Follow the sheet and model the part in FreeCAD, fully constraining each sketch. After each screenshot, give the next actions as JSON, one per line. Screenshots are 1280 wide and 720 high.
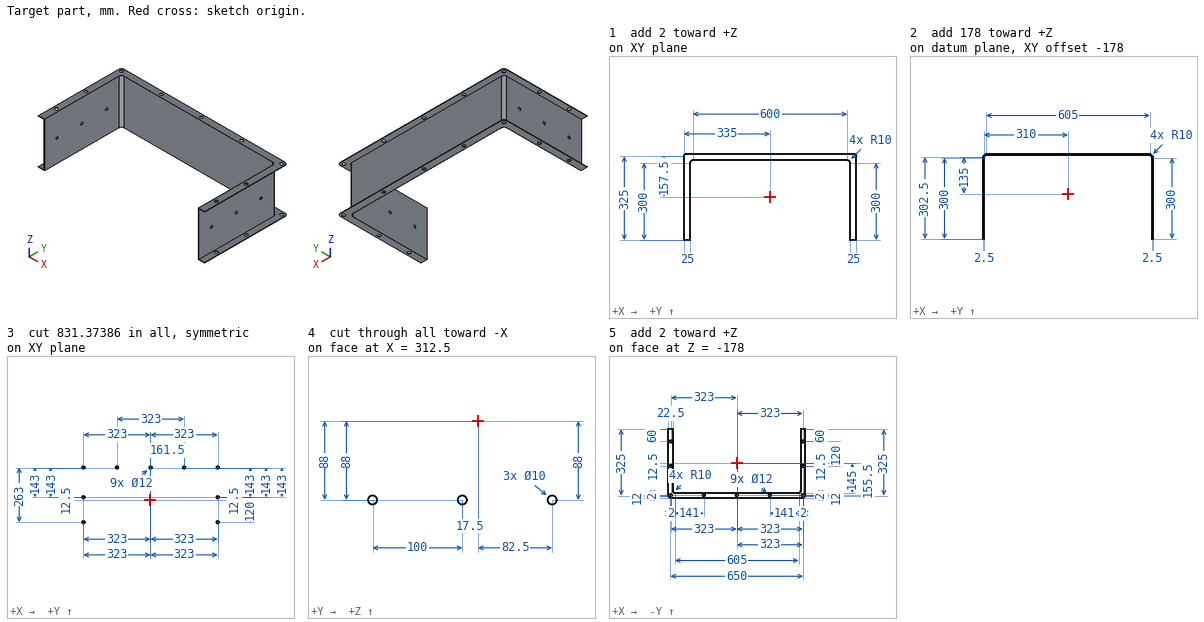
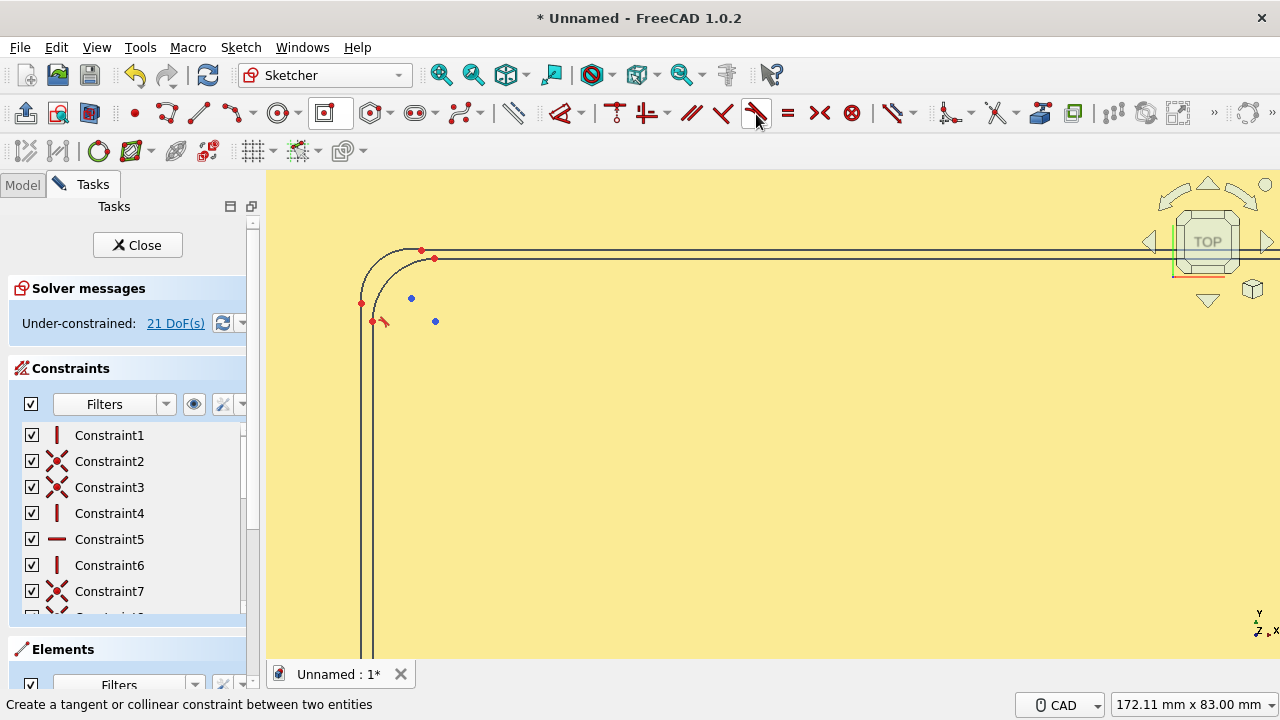
{"action": "scroll", "coordinate": [408, 266], "scroll_direction": "down", "scroll_amount": 9}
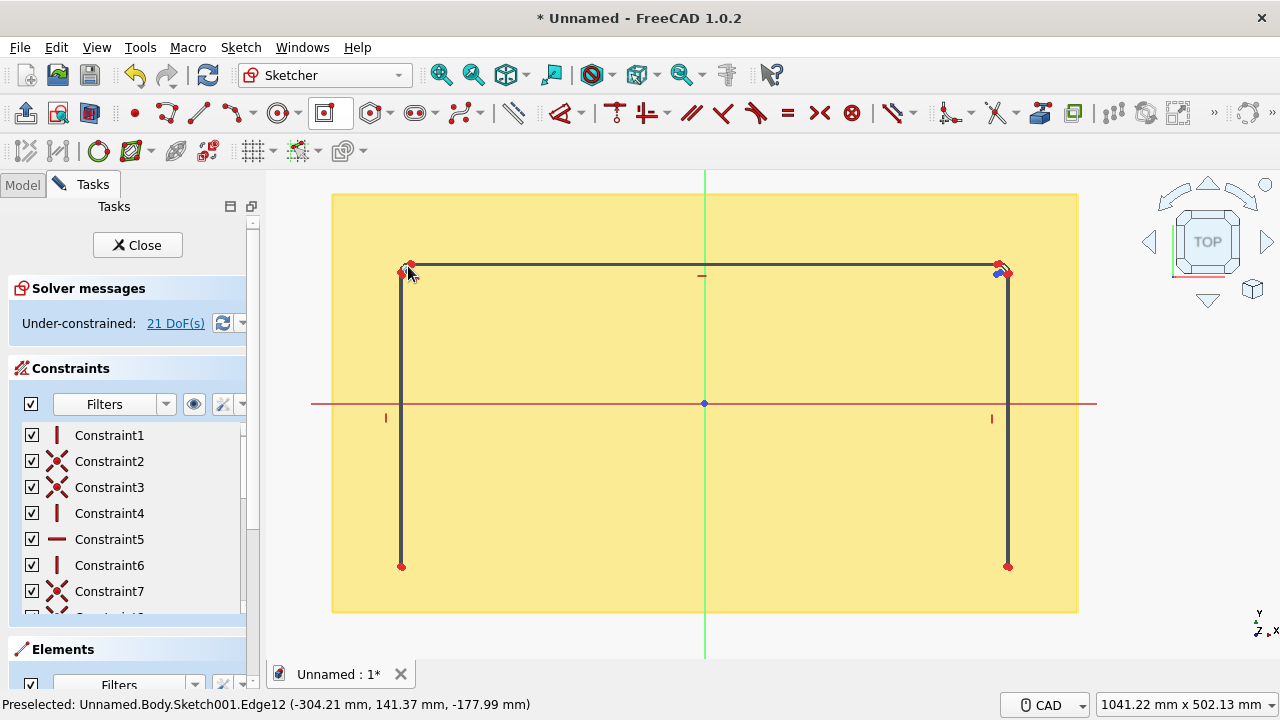
{"action": "scroll", "coordinate": [400, 478], "scroll_direction": "up", "scroll_amount": 10}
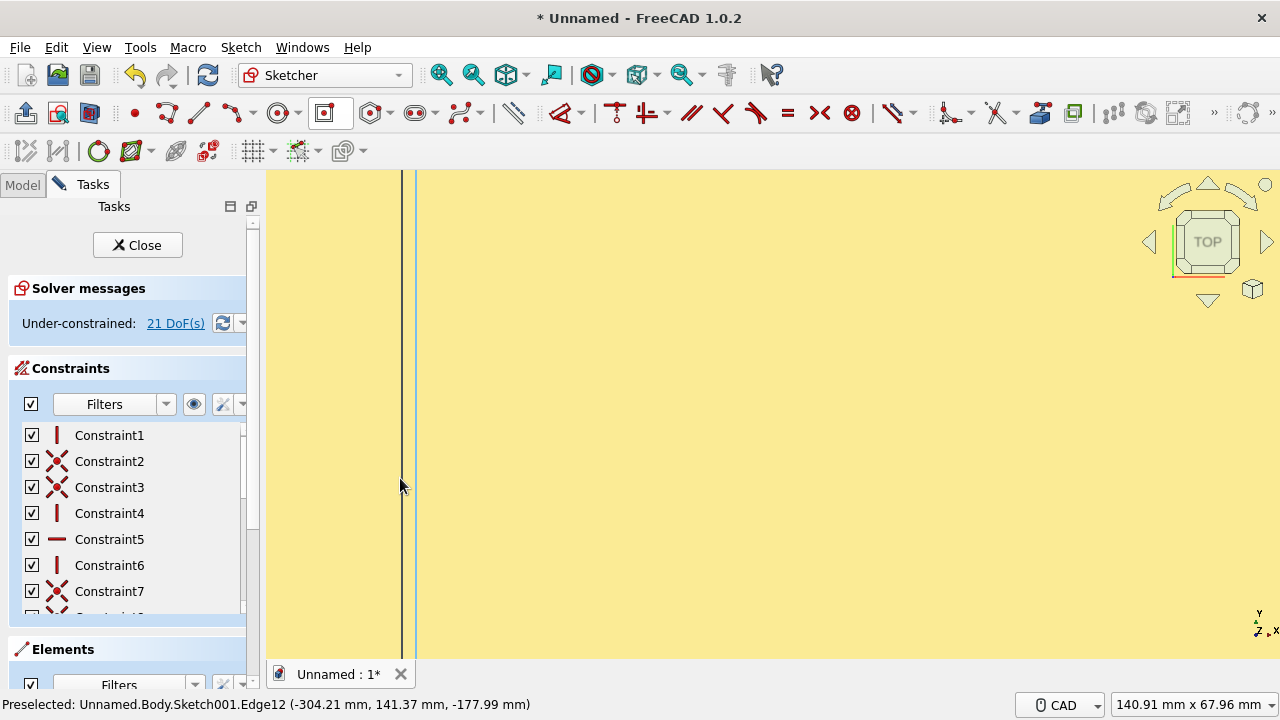
{"action": "left_click", "coordinate": [402, 476]}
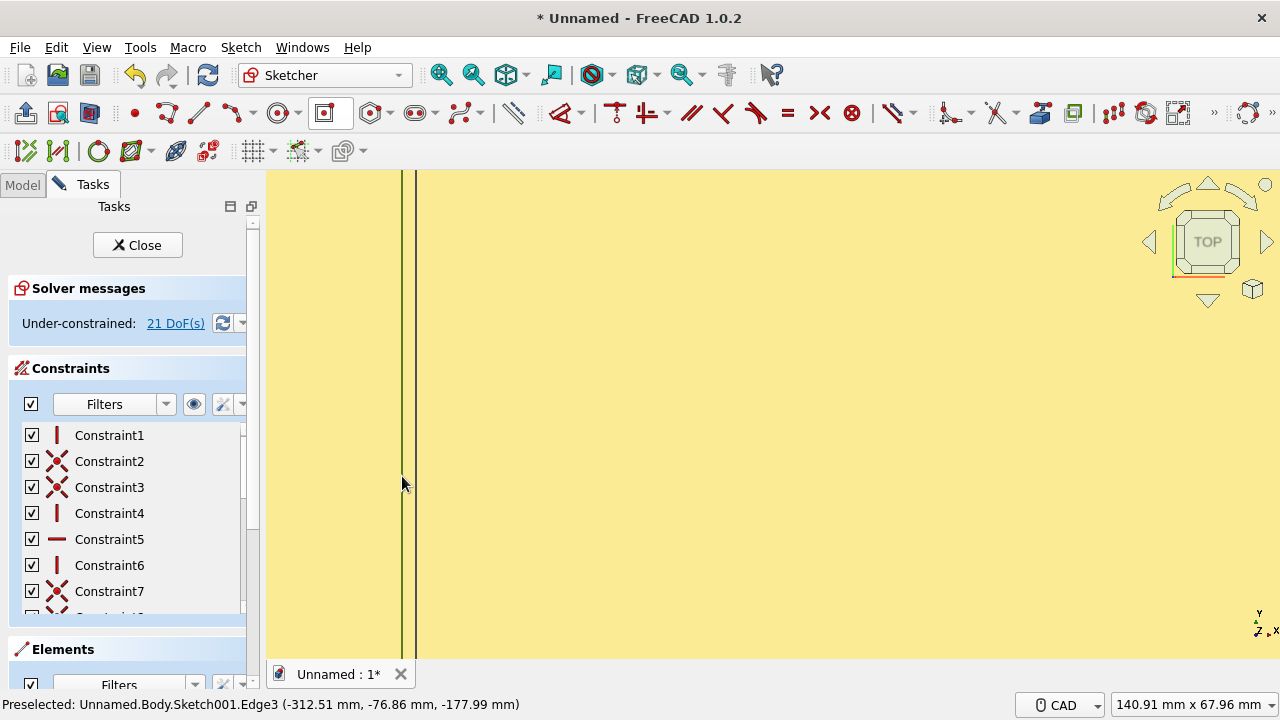
{"action": "scroll", "coordinate": [400, 479], "scroll_direction": "down", "scroll_amount": 10}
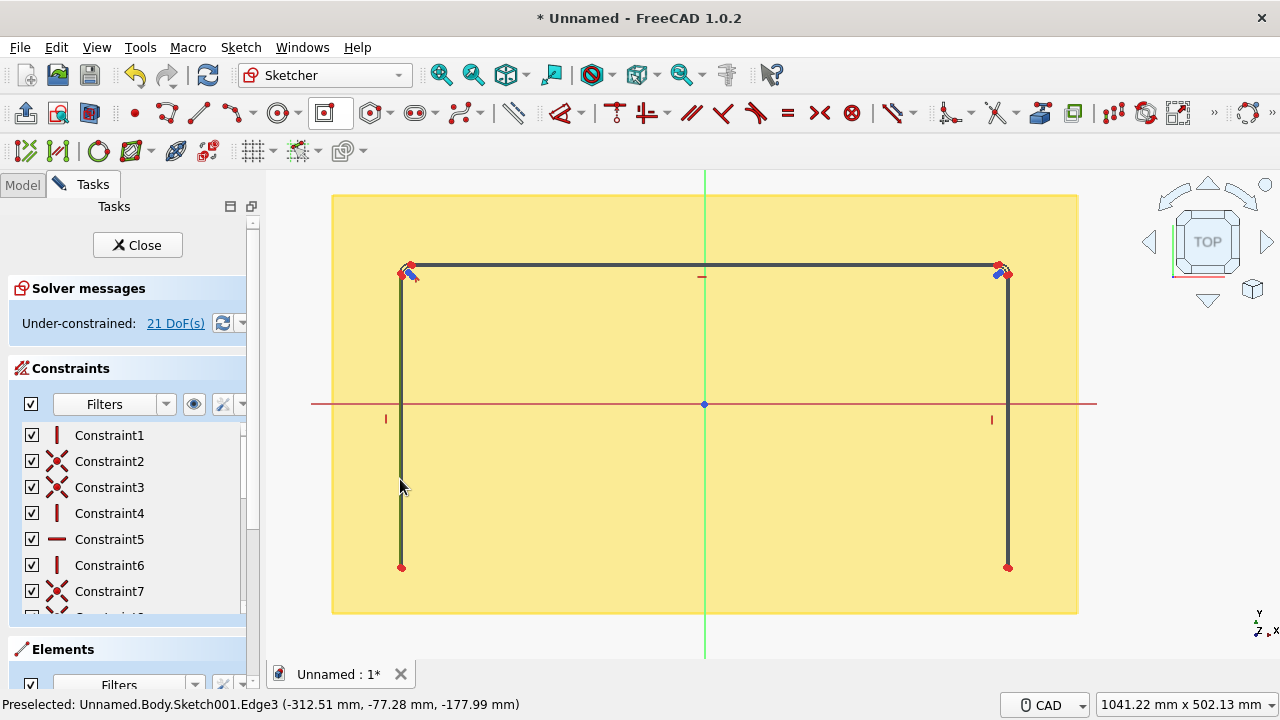
{"action": "scroll", "coordinate": [406, 265], "scroll_direction": "up", "scroll_amount": 8}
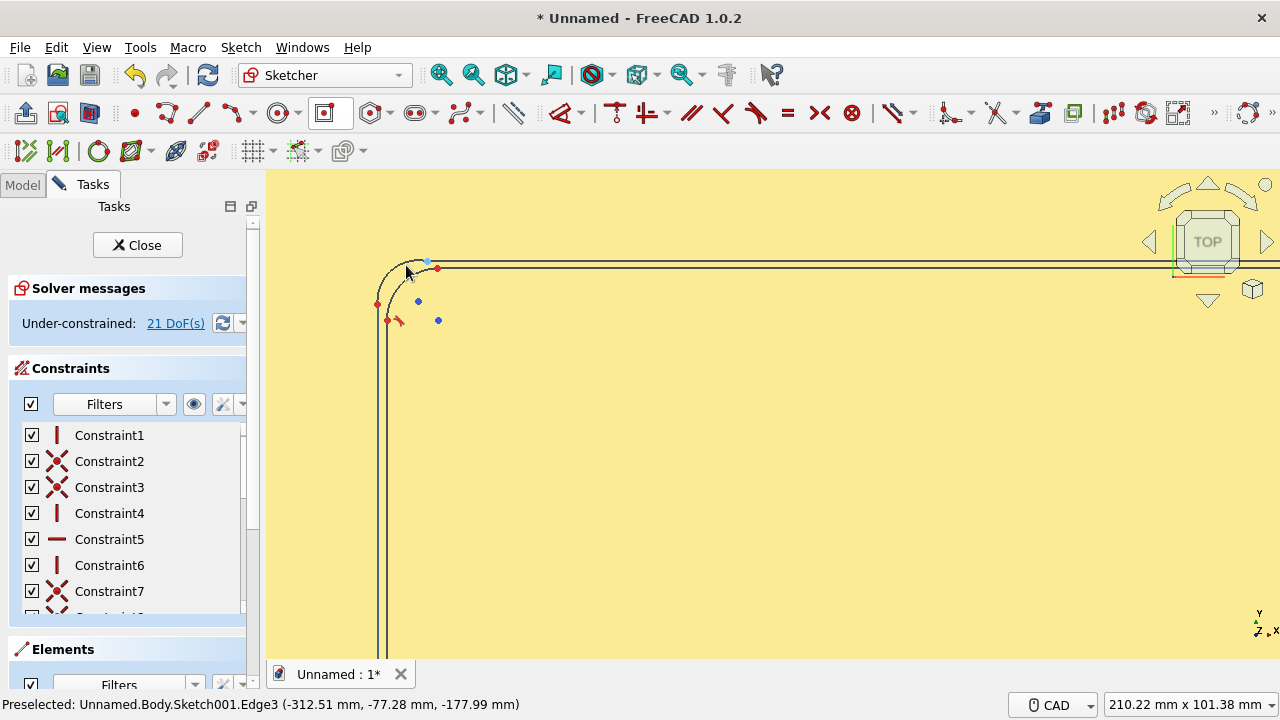
{"action": "left_click", "coordinate": [405, 263]}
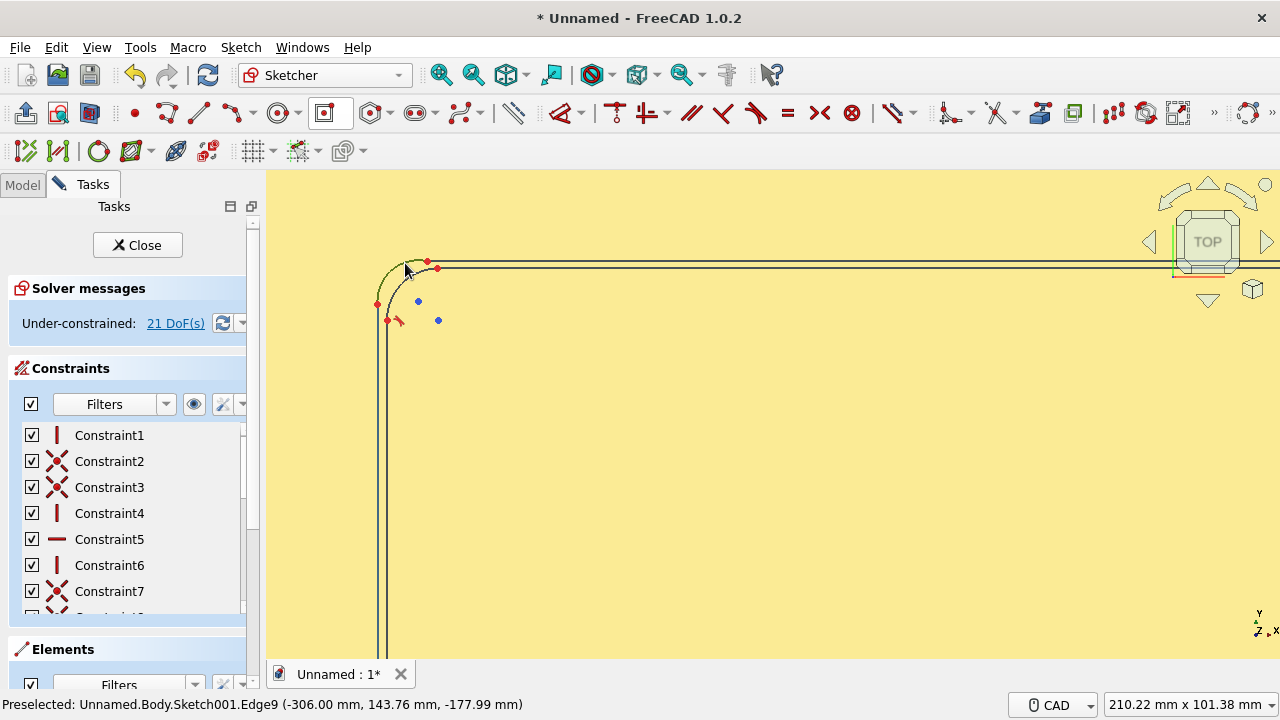
{"action": "left_click", "coordinate": [756, 114]}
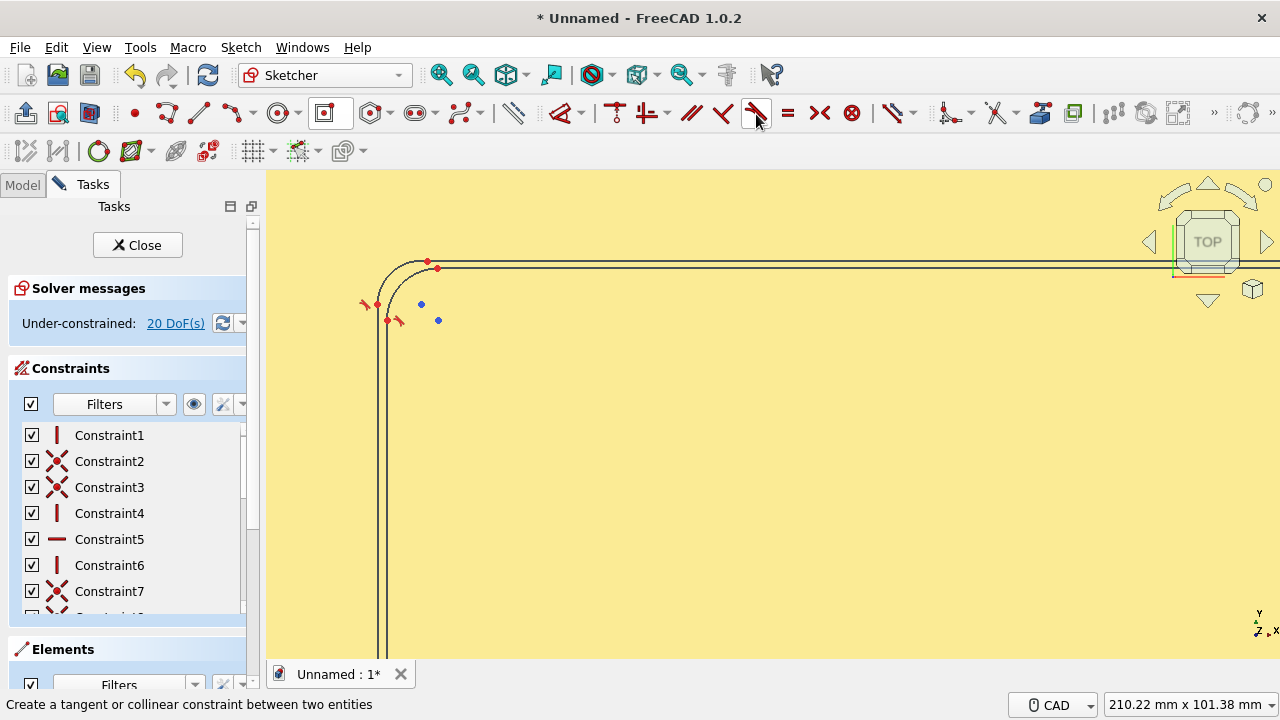
{"action": "scroll", "coordinate": [1011, 261], "scroll_direction": "up", "scroll_amount": 4}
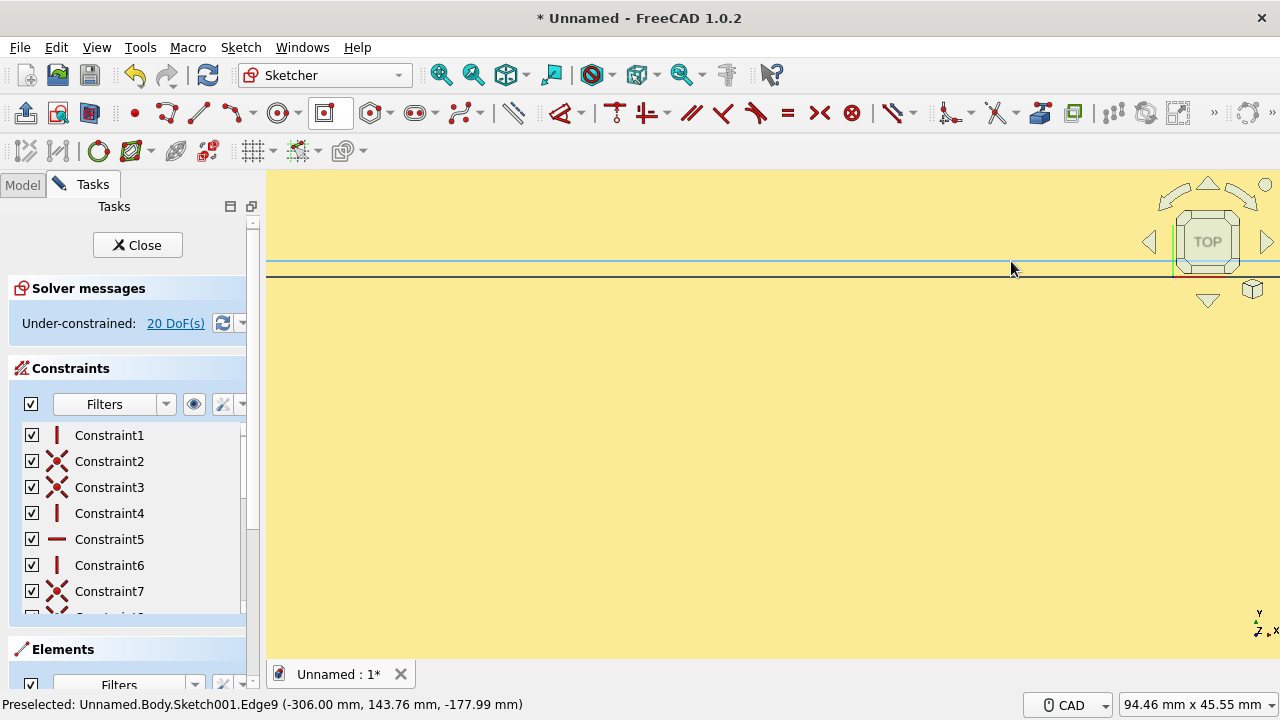
{"action": "left_click", "coordinate": [1009, 261]}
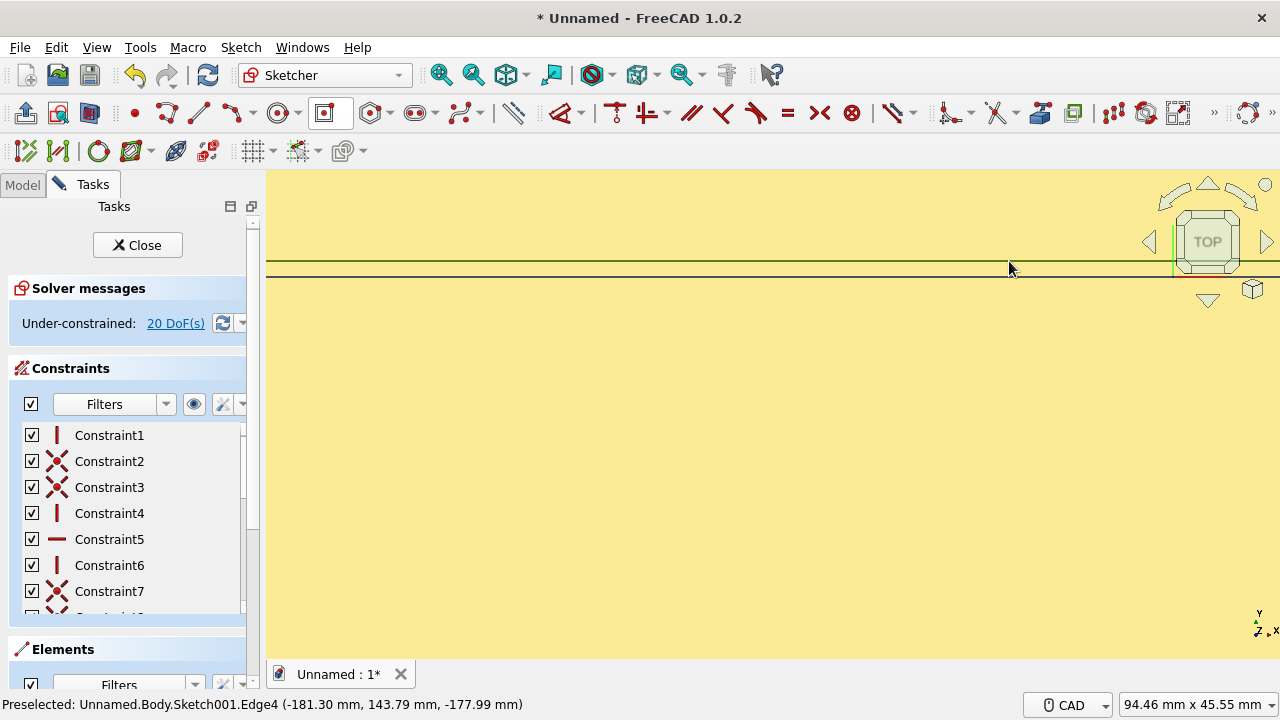
{"action": "scroll", "coordinate": [480, 264], "scroll_direction": "down", "scroll_amount": 12}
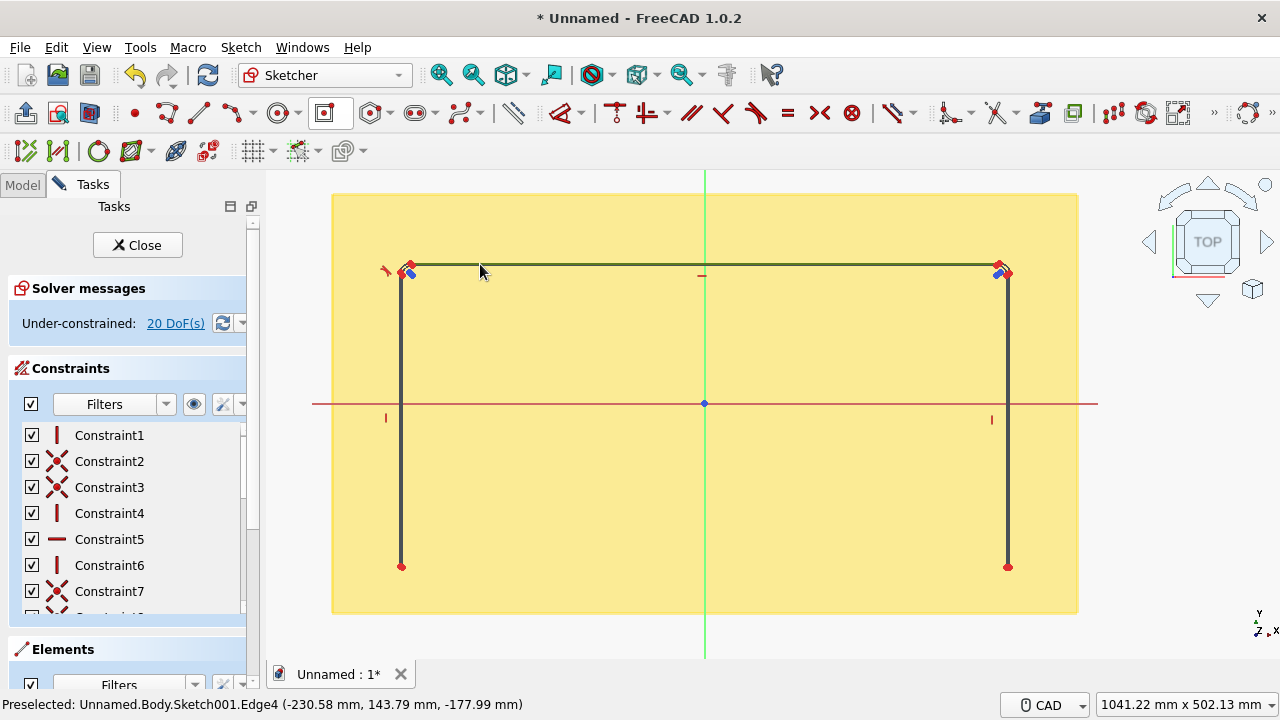
{"action": "scroll", "coordinate": [406, 264], "scroll_direction": "up", "scroll_amount": 9}